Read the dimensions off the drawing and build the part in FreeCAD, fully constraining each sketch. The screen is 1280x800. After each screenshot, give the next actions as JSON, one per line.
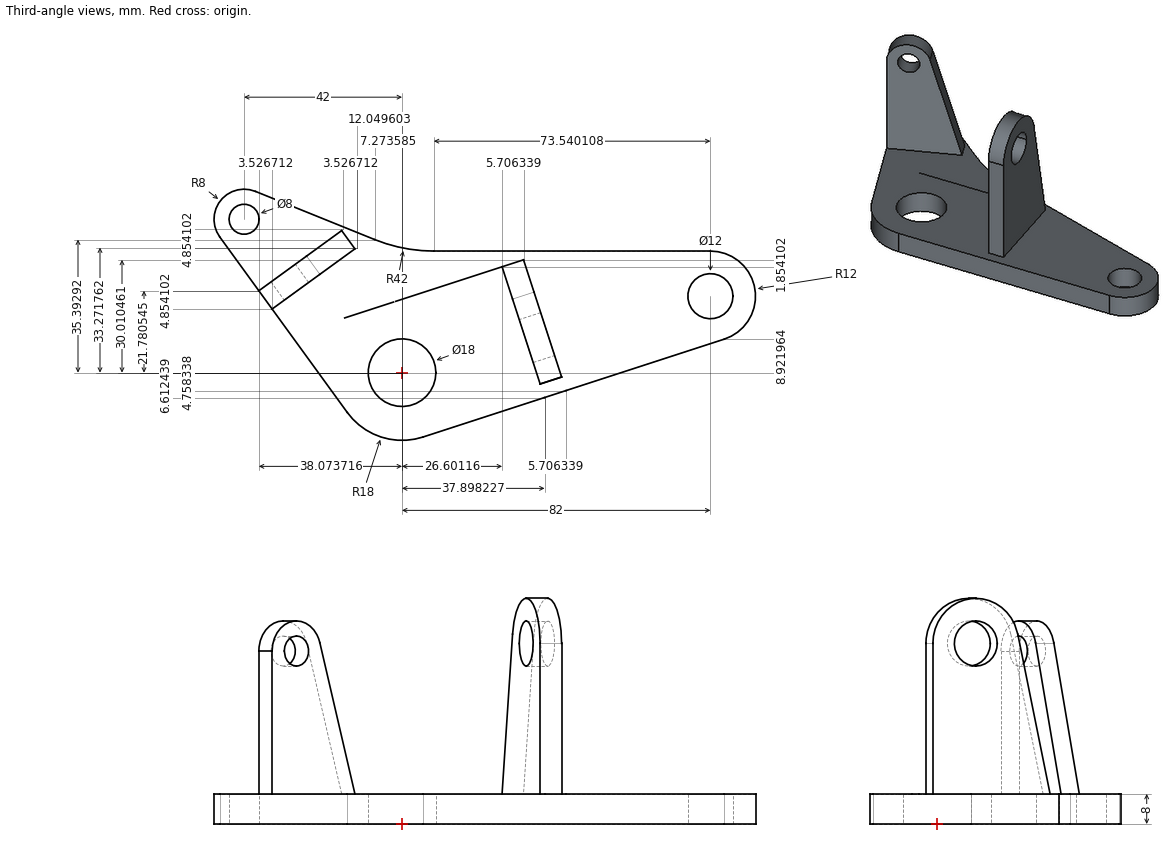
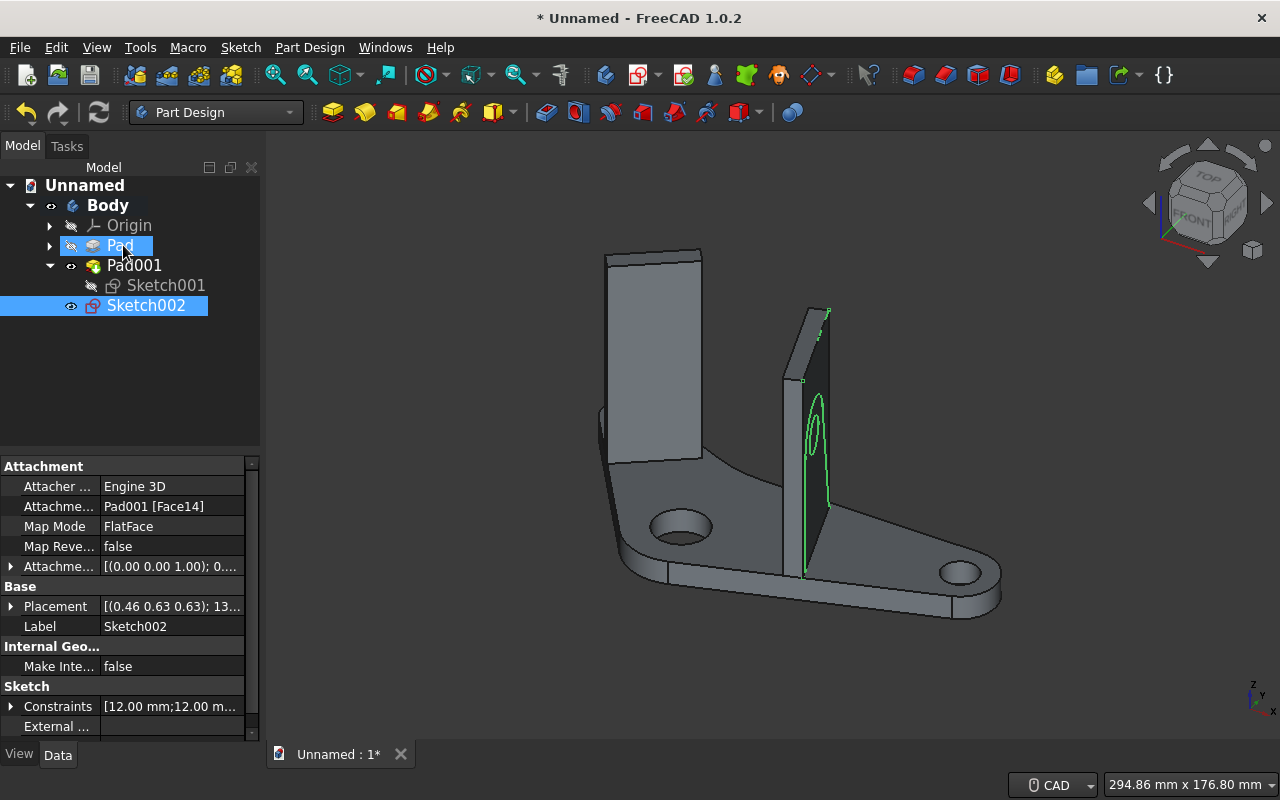
{"action": "left_click", "coordinate": [548, 112]}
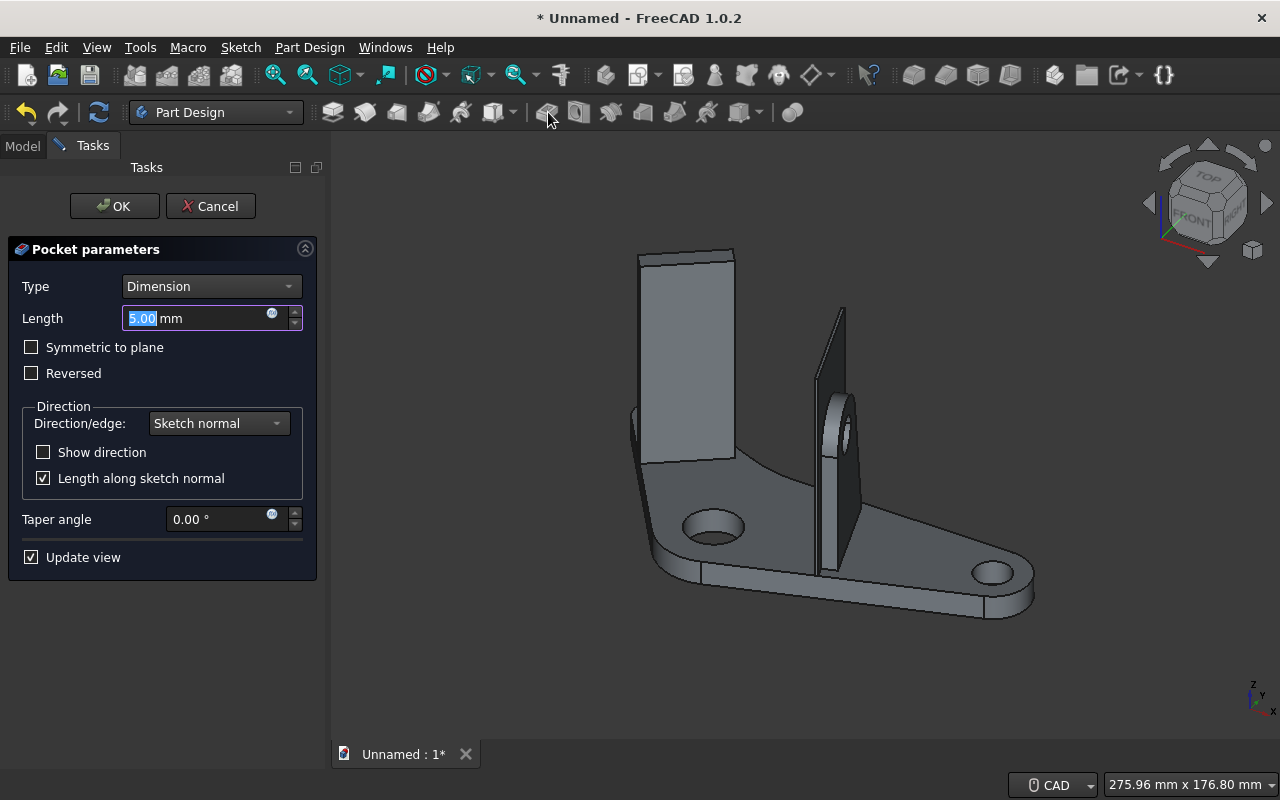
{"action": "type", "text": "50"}
{"action": "key", "text": "Tab"}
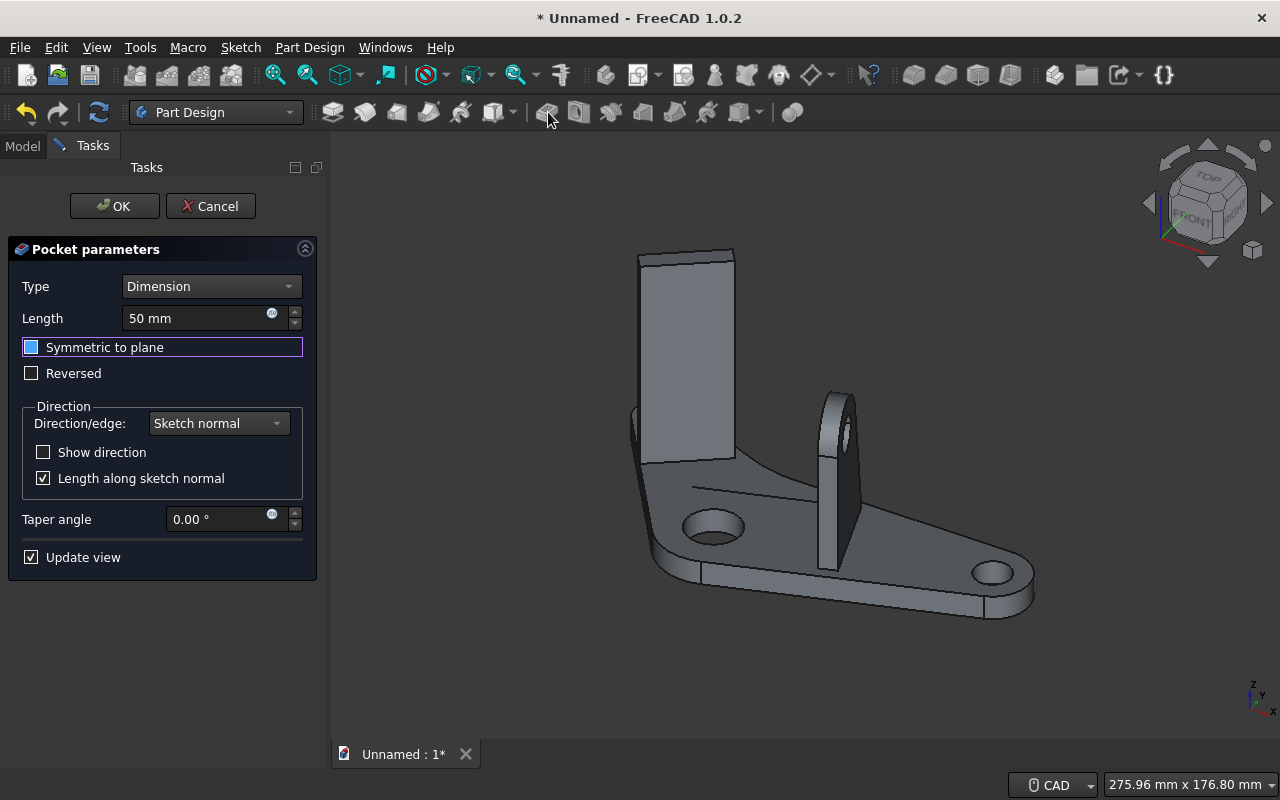
{"action": "left_click", "coordinate": [115, 206]}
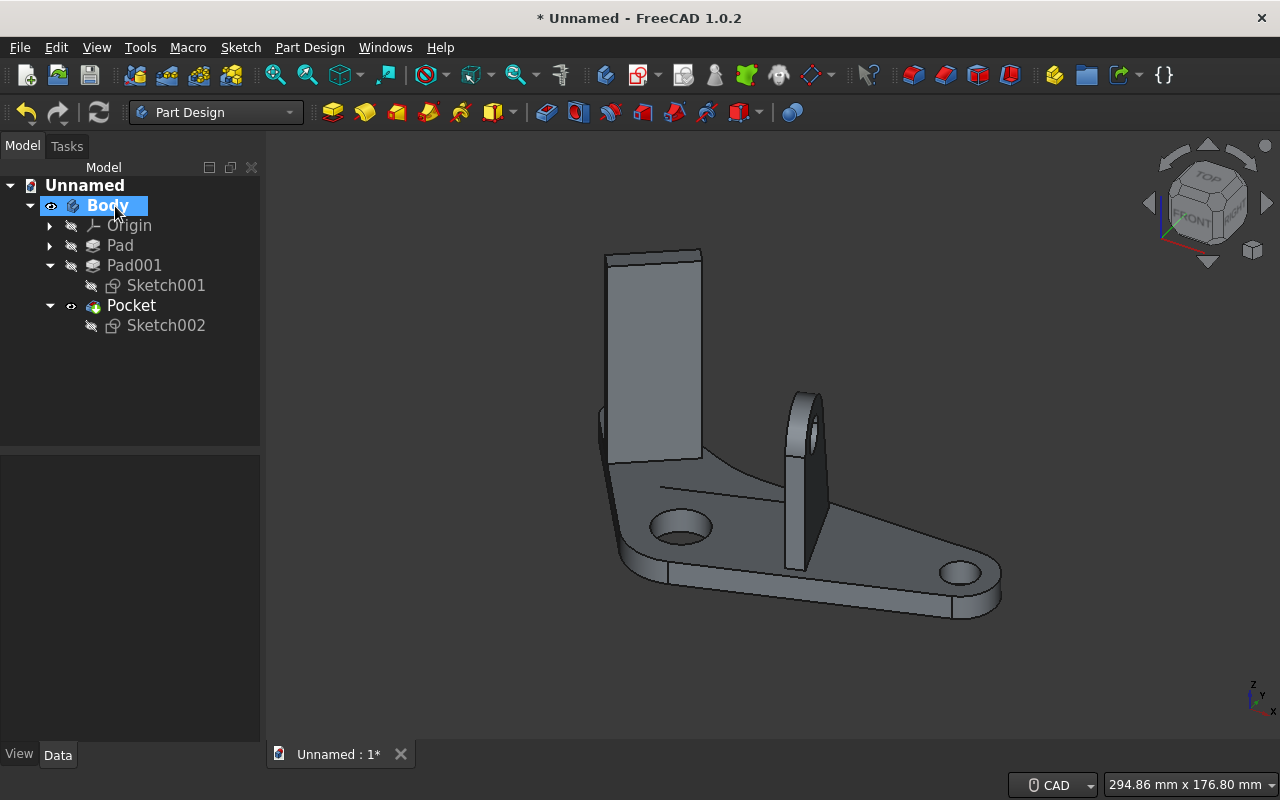
{"action": "key", "text": "4"}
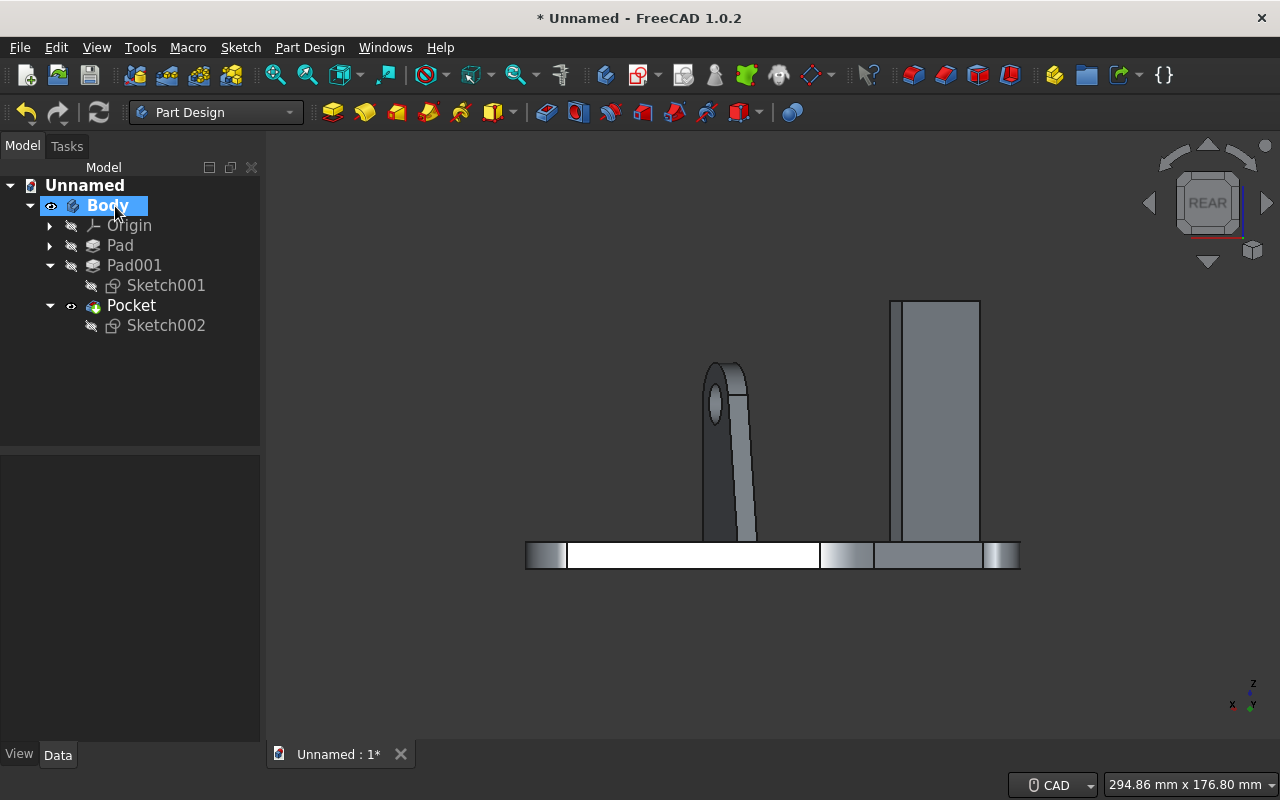
{"action": "left_click", "coordinate": [941, 351]}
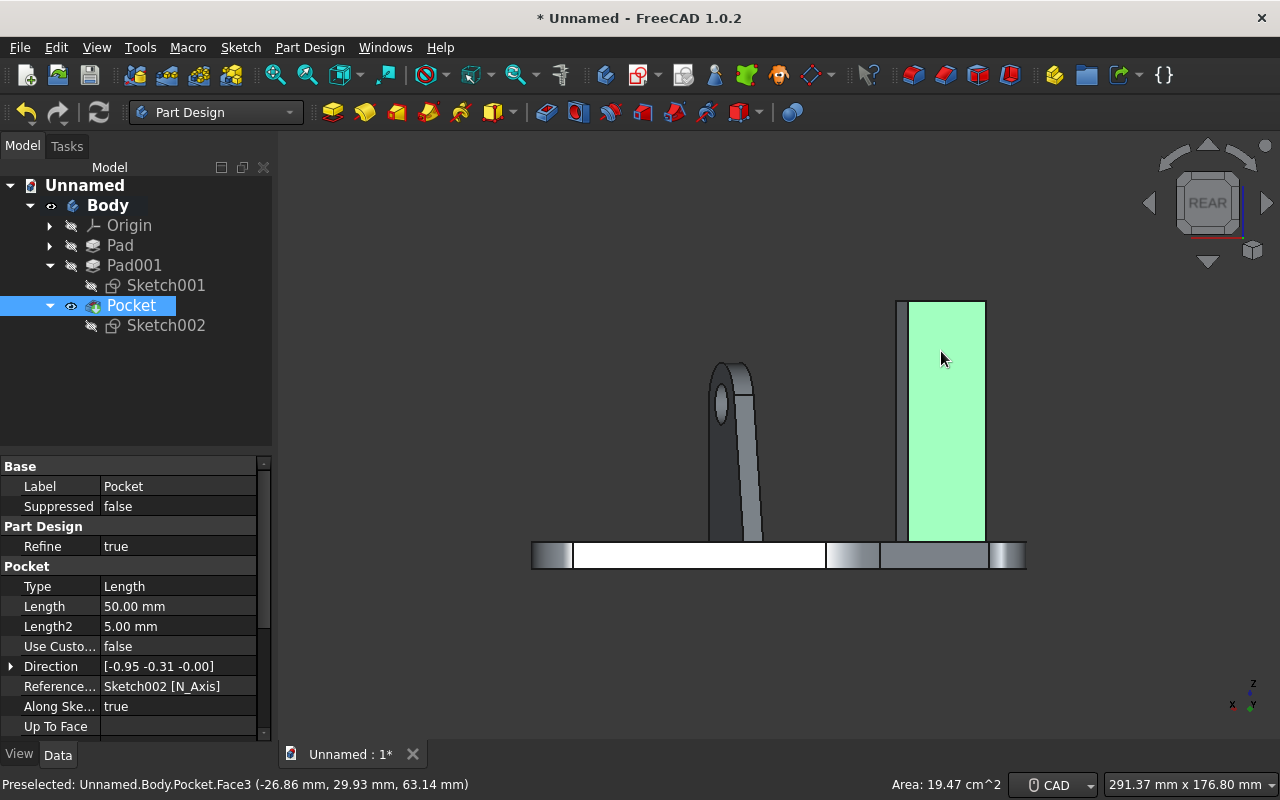
{"action": "left_click", "coordinate": [638, 76]}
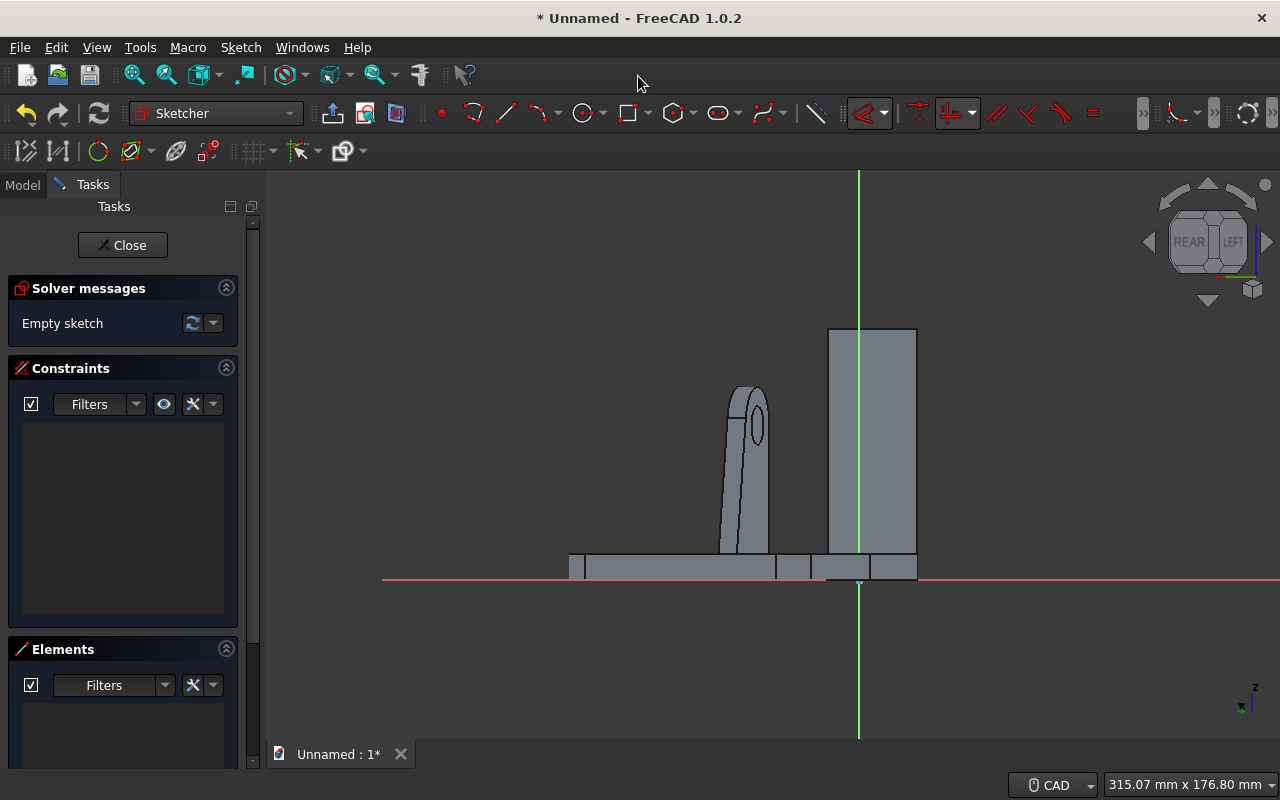
{"action": "left_click", "coordinate": [398, 114]}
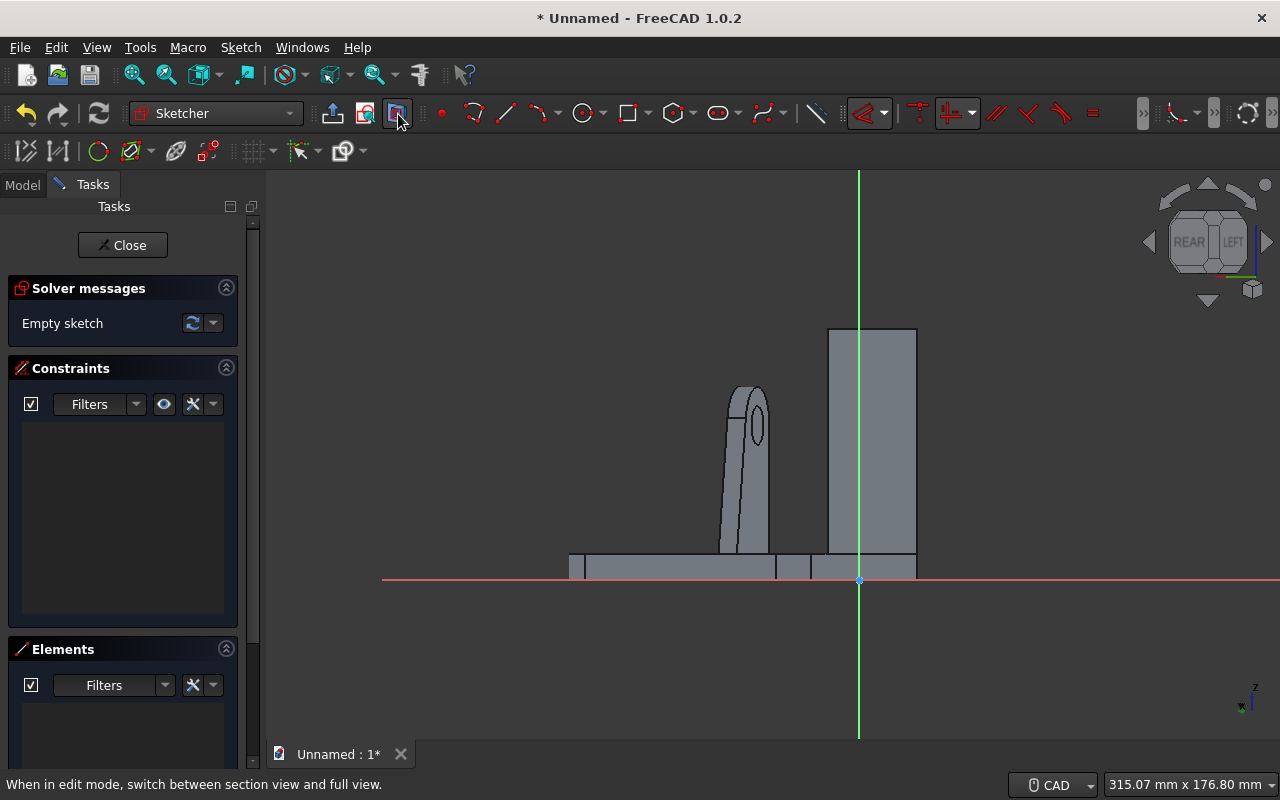
{"action": "scroll", "coordinate": [1115, 455], "scroll_direction": "up", "scroll_amount": 2}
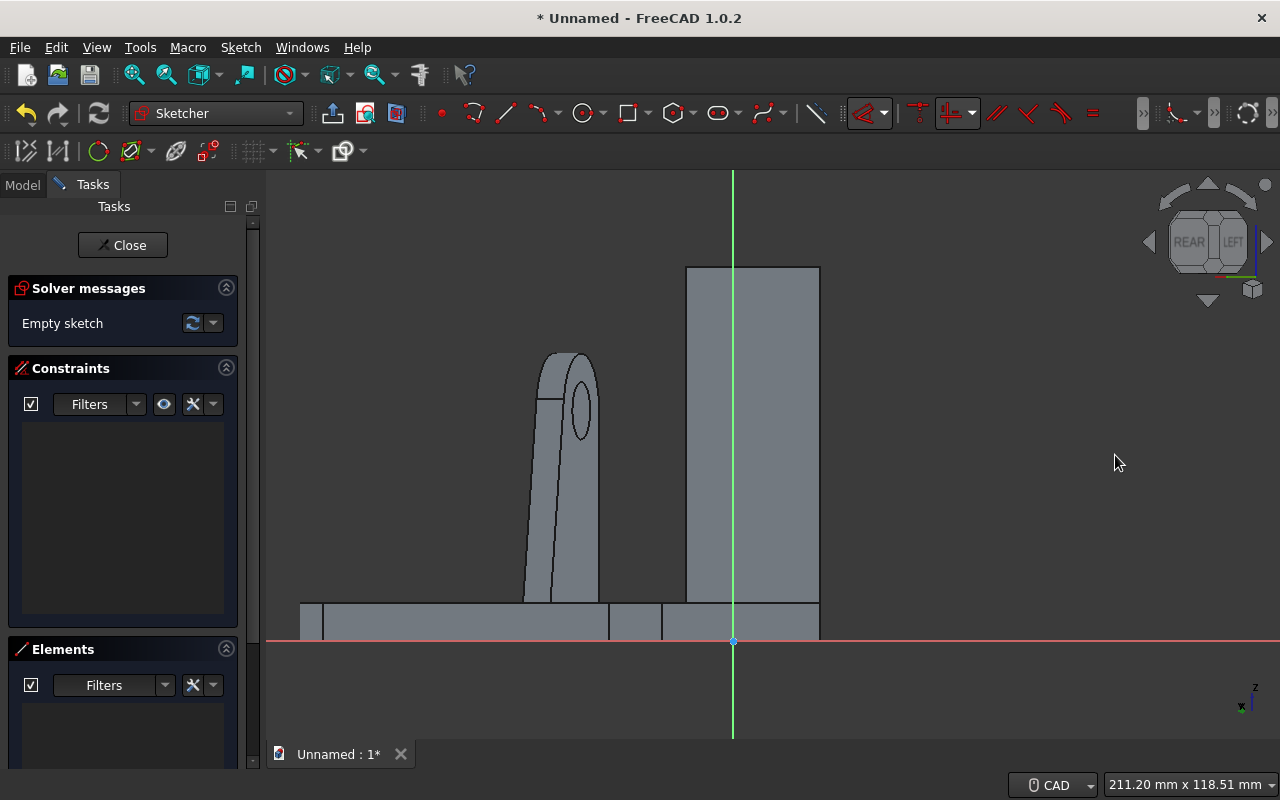
{"action": "left_click", "coordinate": [474, 114]}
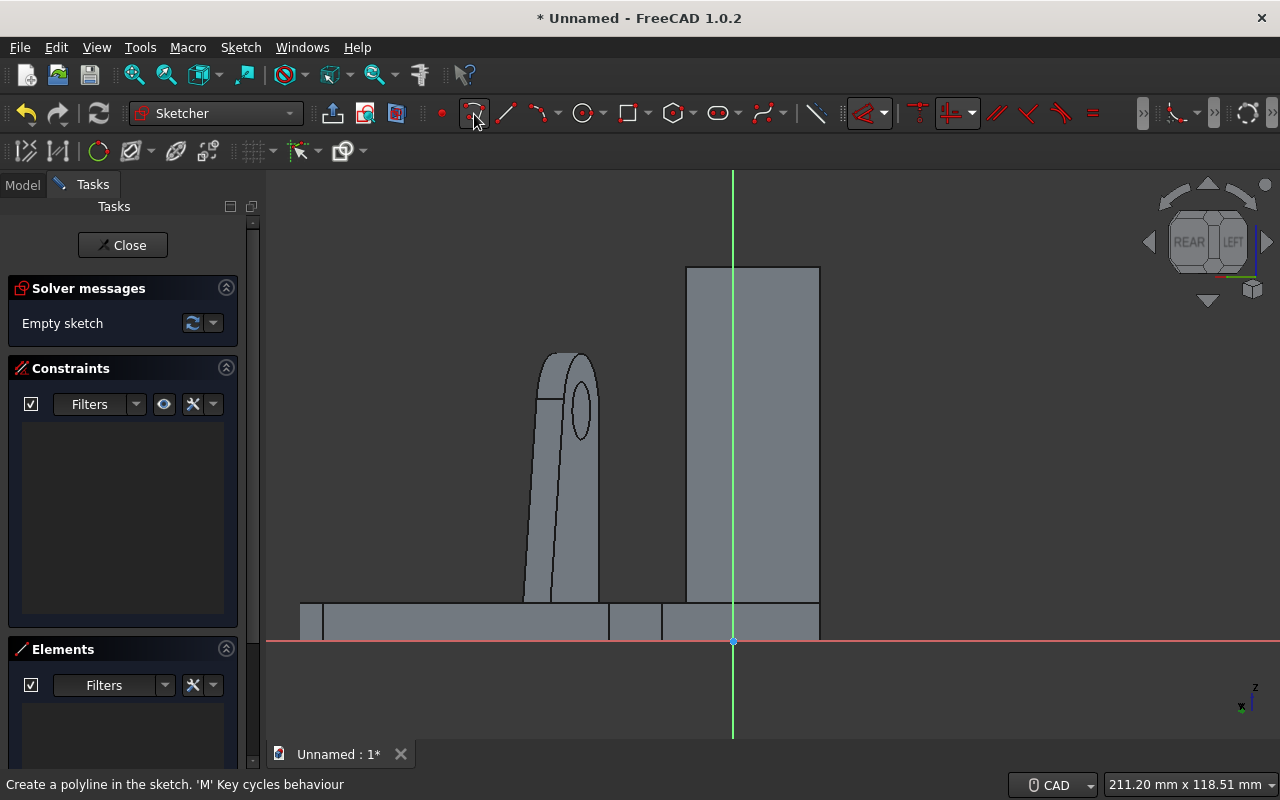
{"action": "left_click", "coordinate": [820, 420]}
{"action": "left_click", "coordinate": [820, 267]}
{"action": "left_click", "coordinate": [686, 267]}
{"action": "left_click", "coordinate": [686, 603]}